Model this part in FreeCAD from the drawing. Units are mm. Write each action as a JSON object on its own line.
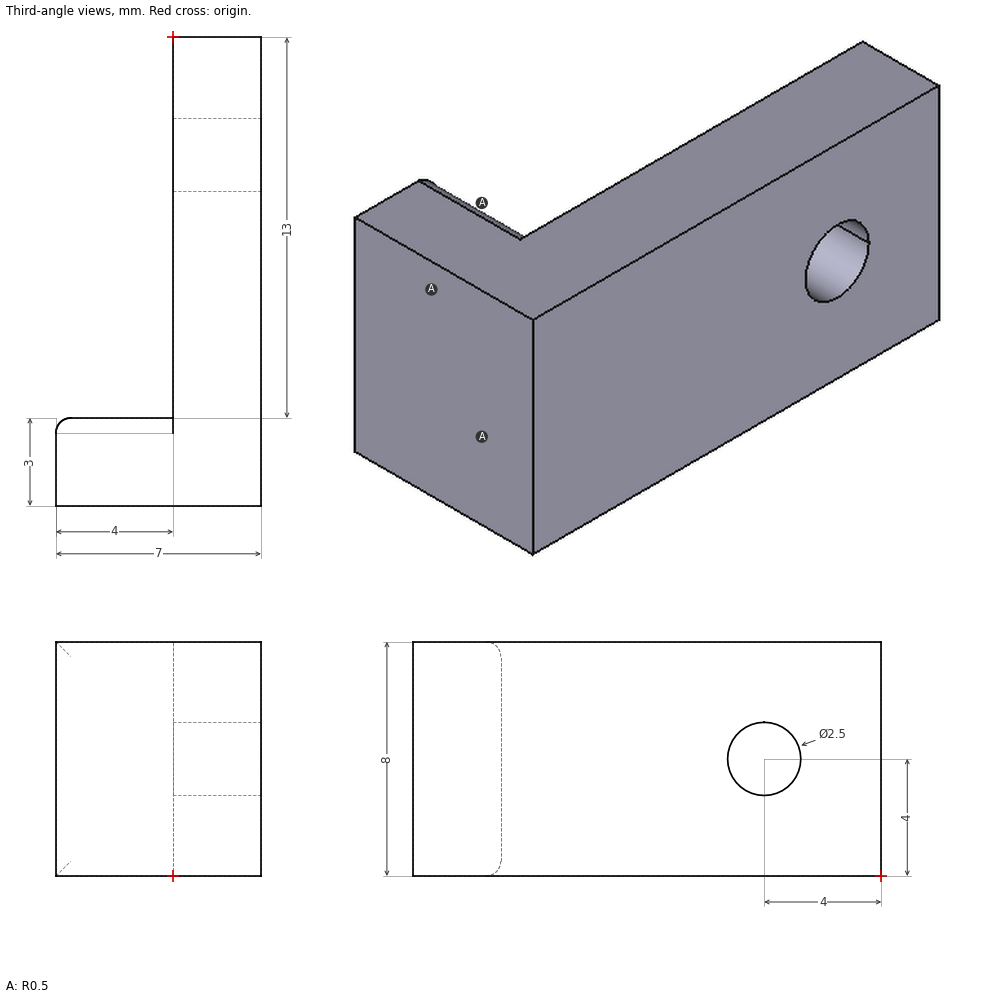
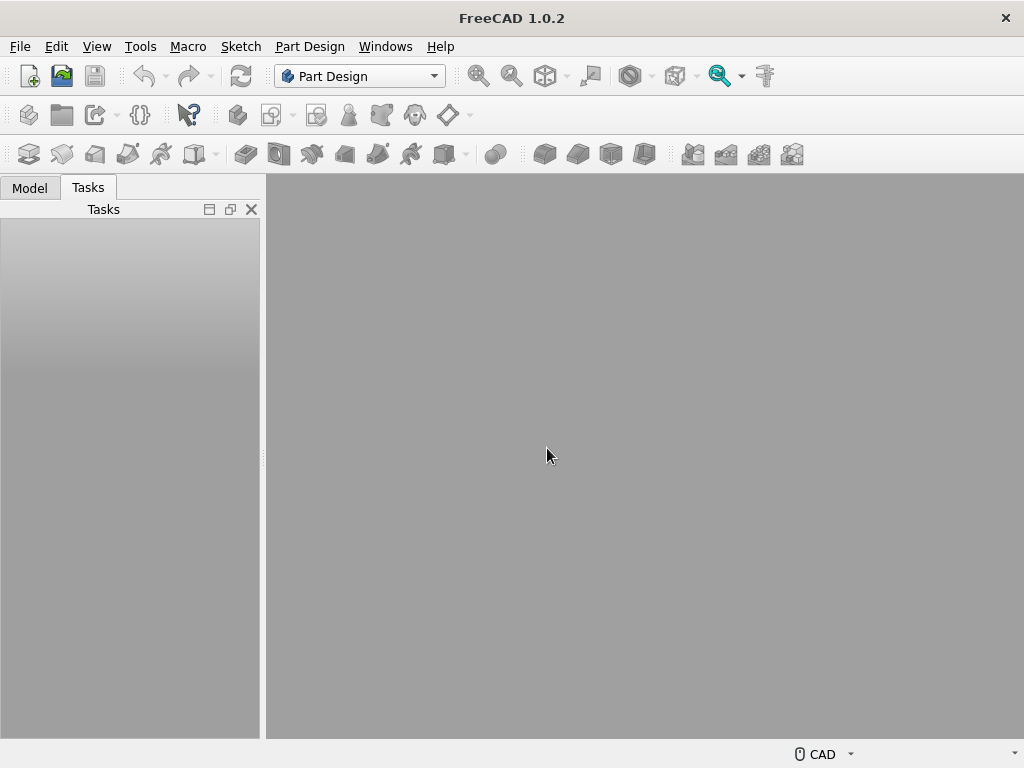
{"action": "left_click", "coordinate": [29, 76]}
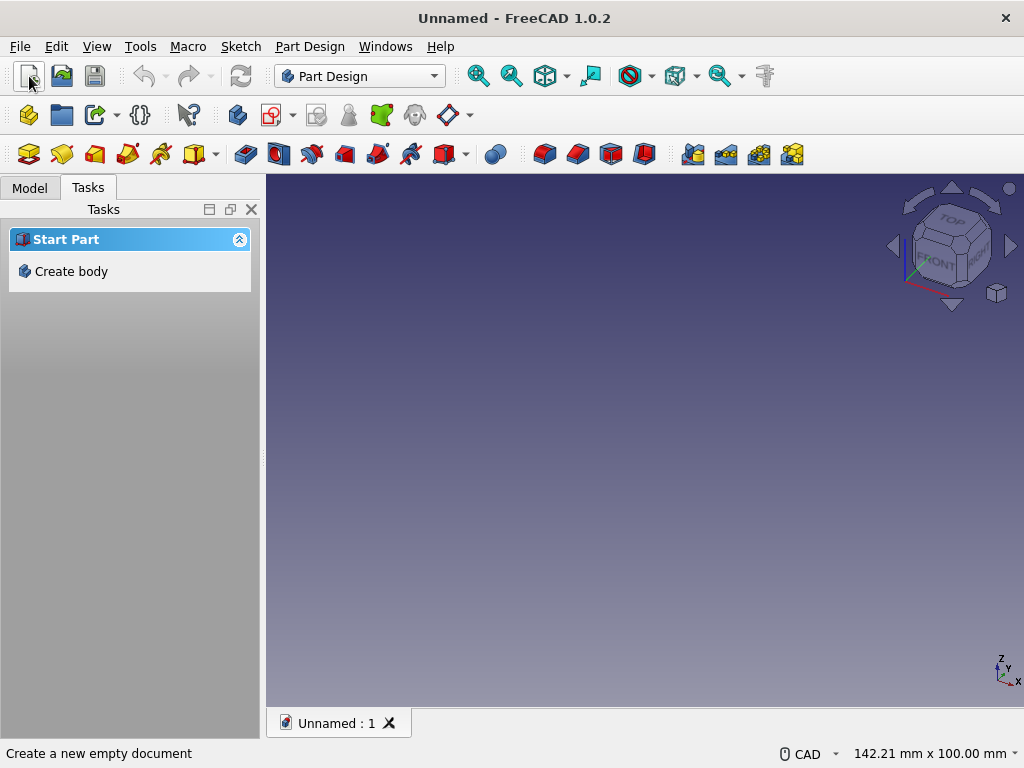
{"action": "left_click", "coordinate": [270, 116]}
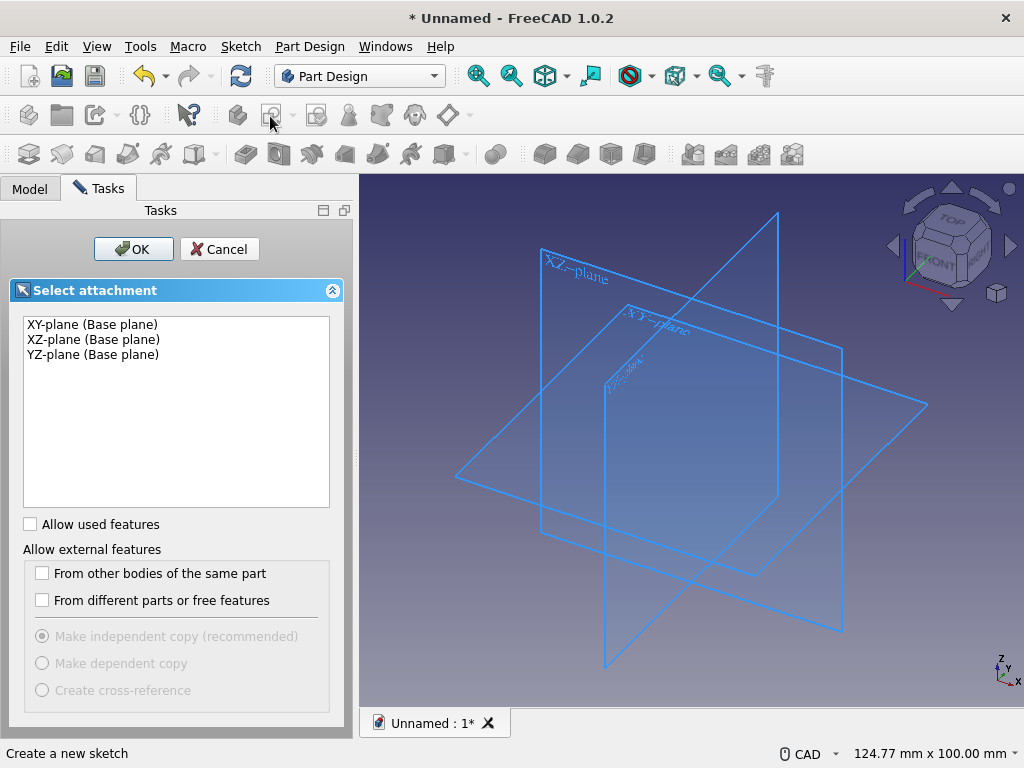
{"action": "left_click", "coordinate": [84, 324]}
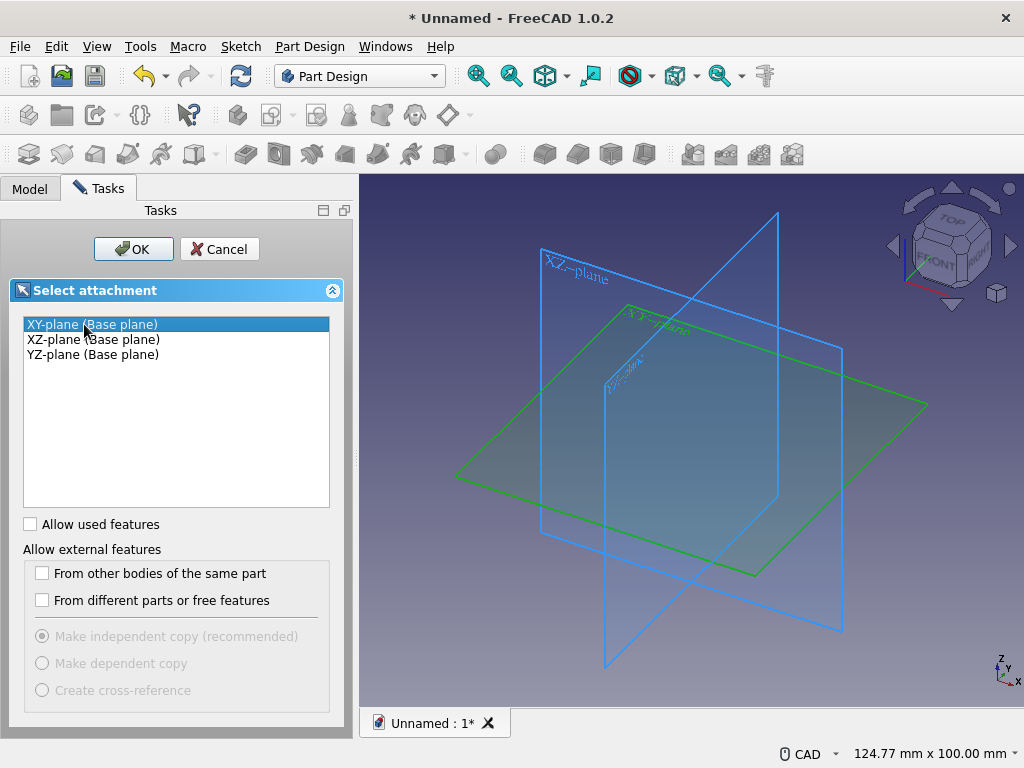
{"action": "left_click", "coordinate": [134, 249]}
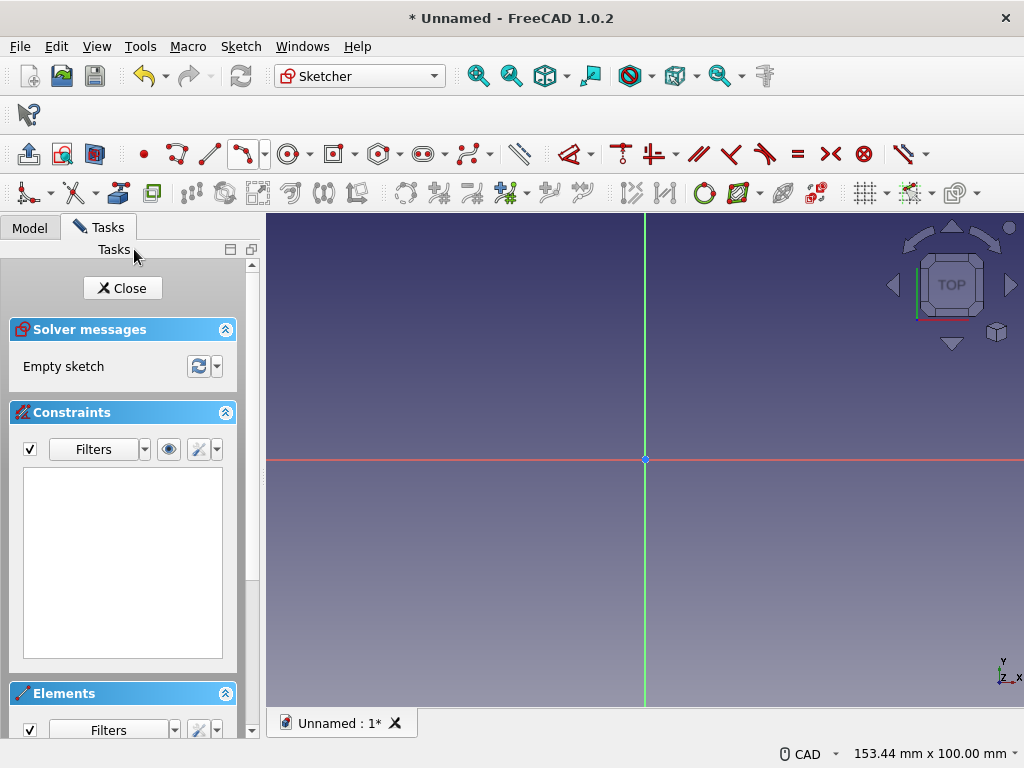
{"action": "scroll", "coordinate": [664, 512], "scroll_direction": "up", "scroll_amount": 7}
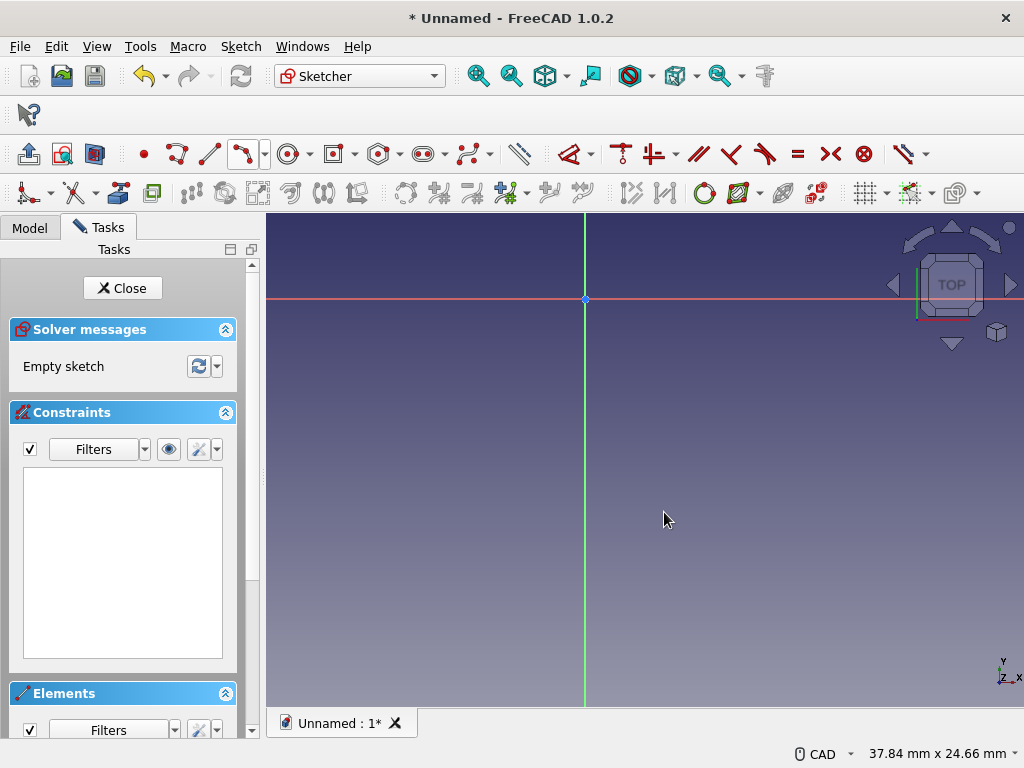
{"action": "left_click", "coordinate": [177, 154]}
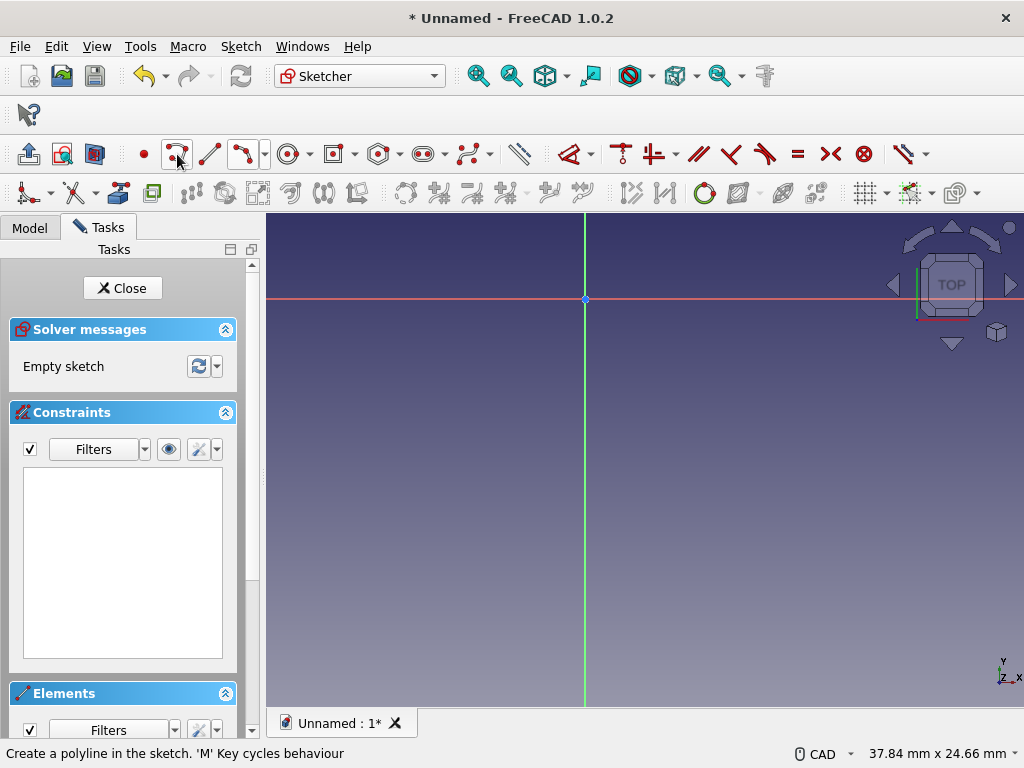
{"action": "left_click", "coordinate": [585, 299]}
{"action": "left_click", "coordinate": [576, 560]}
{"action": "left_click", "coordinate": [505, 560]}
{"action": "left_click", "coordinate": [505, 620]}
{"action": "left_click", "coordinate": [645, 620]}
{"action": "left_click", "coordinate": [645, 308]}
{"action": "left_click", "coordinate": [585, 299]}
{"action": "key", "text": "Escape"}
{"action": "key", "text": "Escape"}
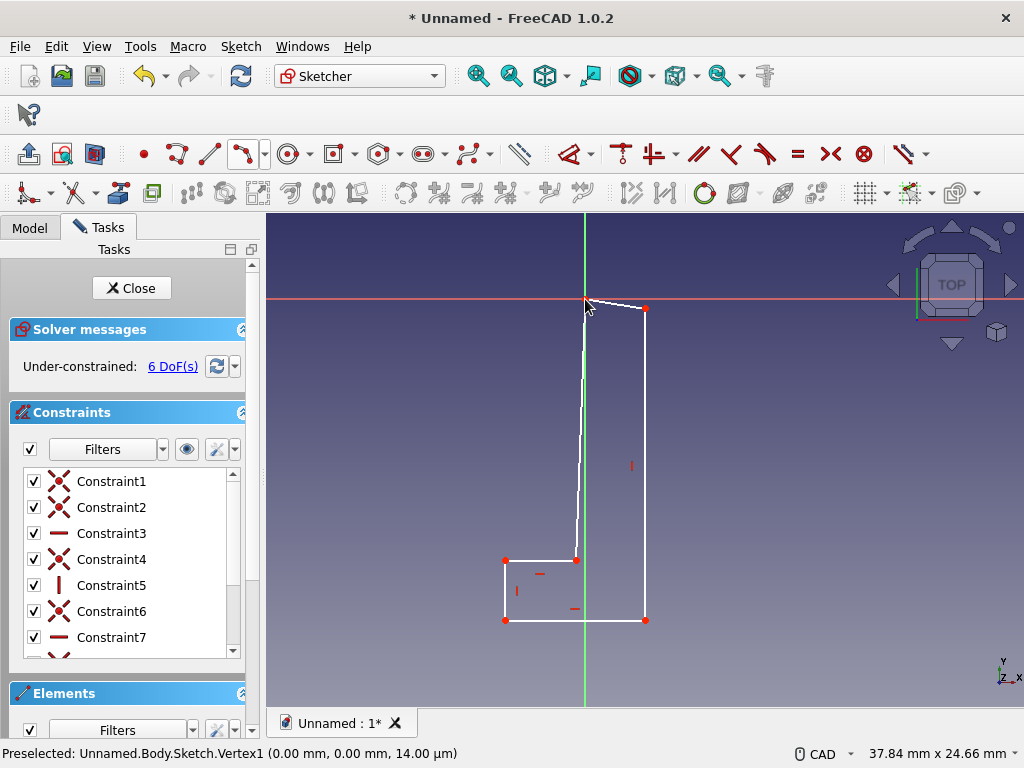
{"action": "left_click", "coordinate": [583, 378]}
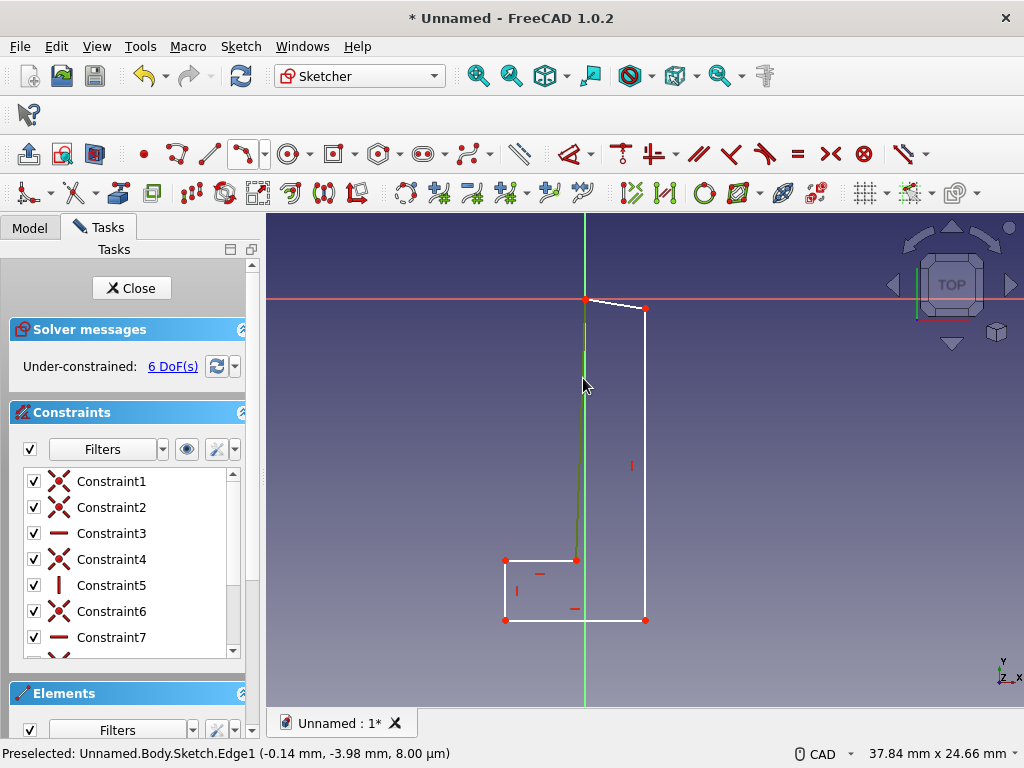
{"action": "left_click", "coordinate": [676, 154]}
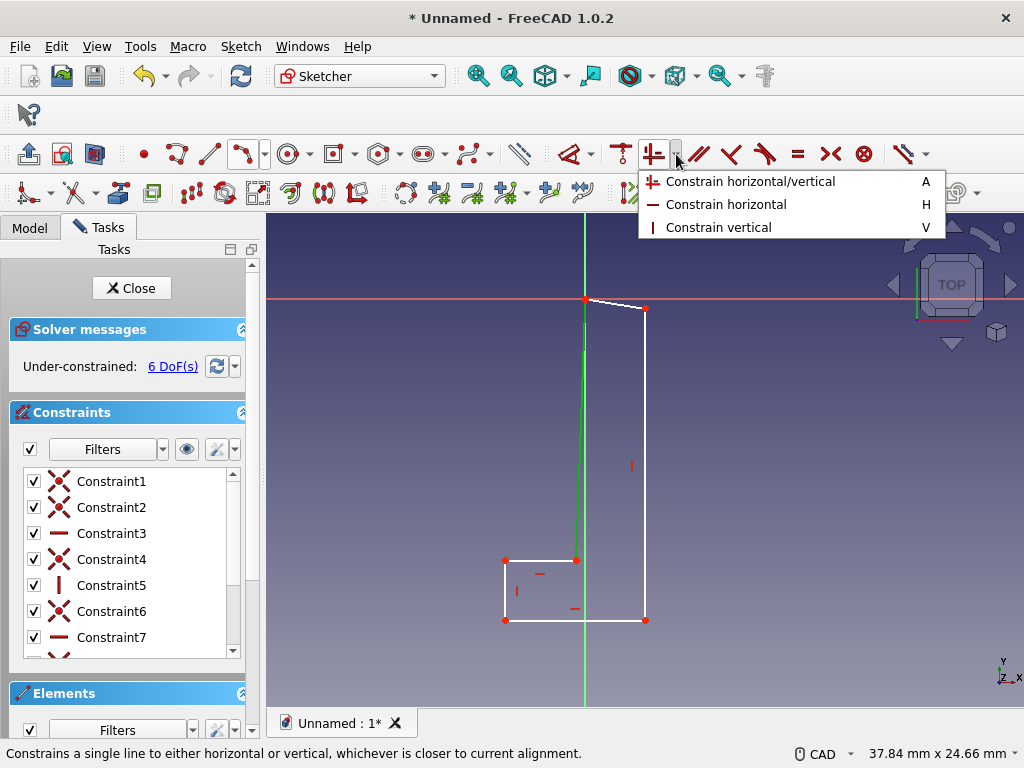
{"action": "left_click", "coordinate": [792, 228]}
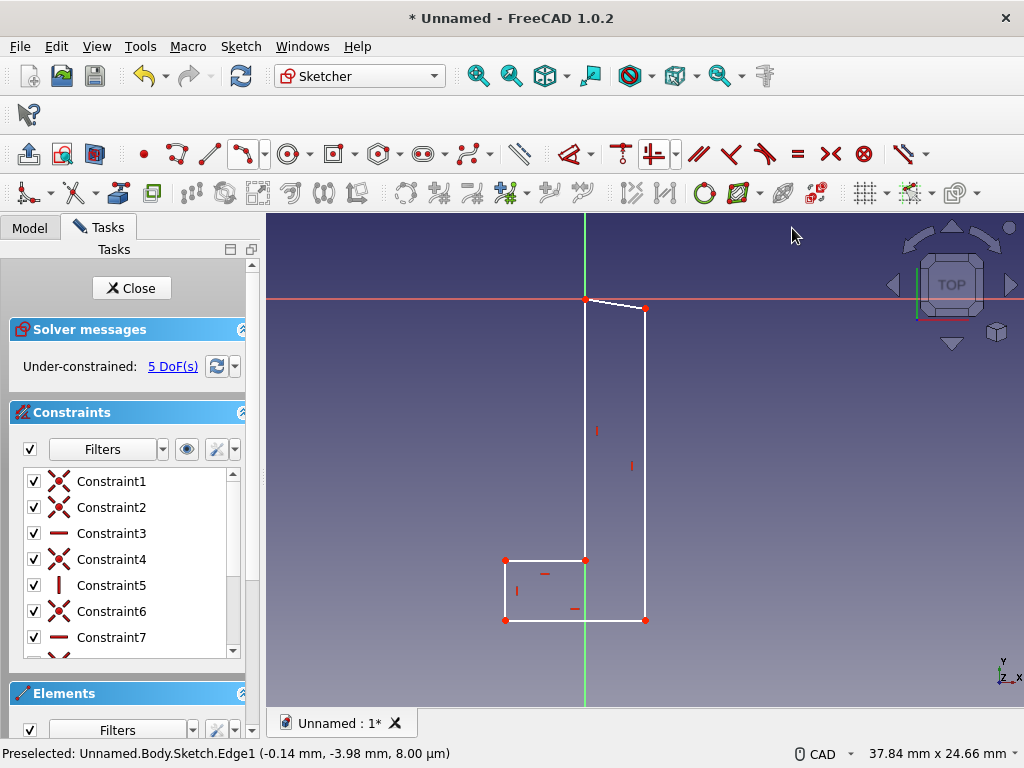
{"action": "left_click", "coordinate": [603, 302]}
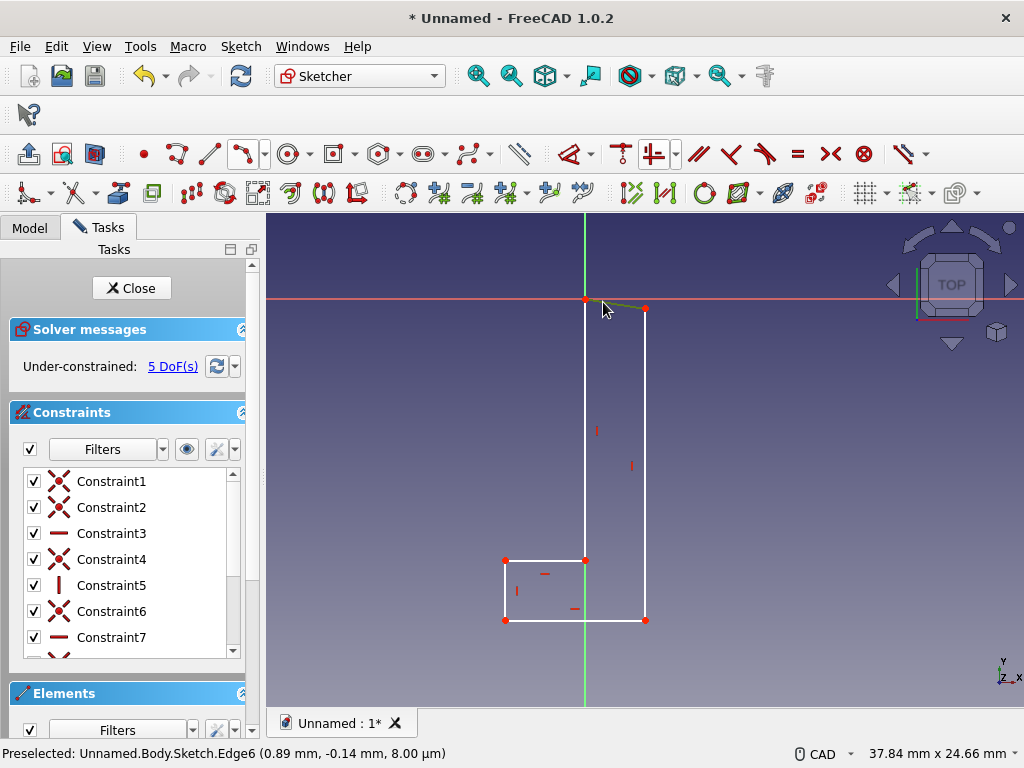
{"action": "key", "text": "h"}